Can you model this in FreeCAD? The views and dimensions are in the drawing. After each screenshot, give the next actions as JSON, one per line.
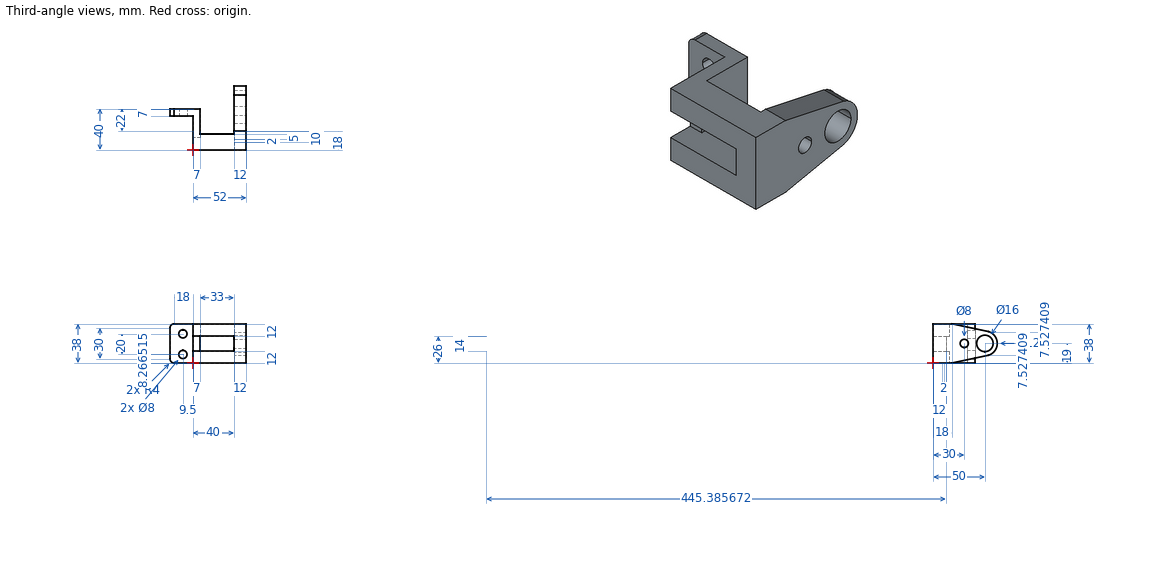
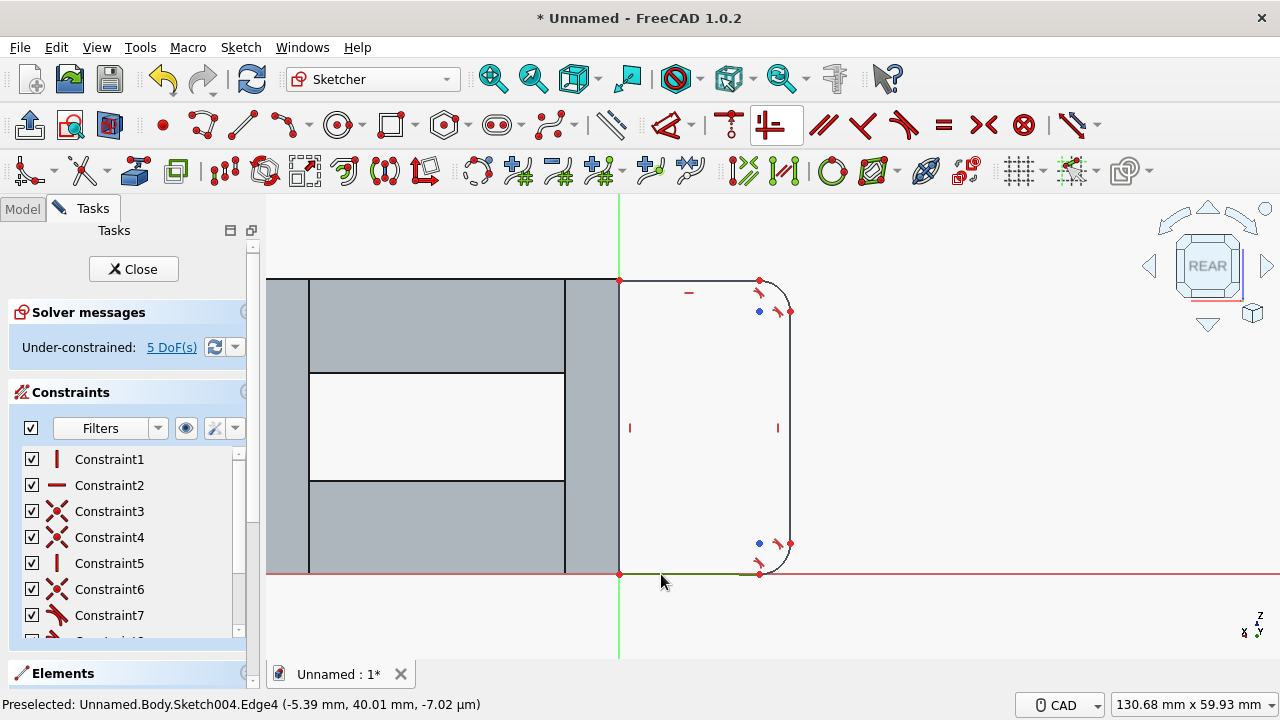
{"action": "key", "text": "h"}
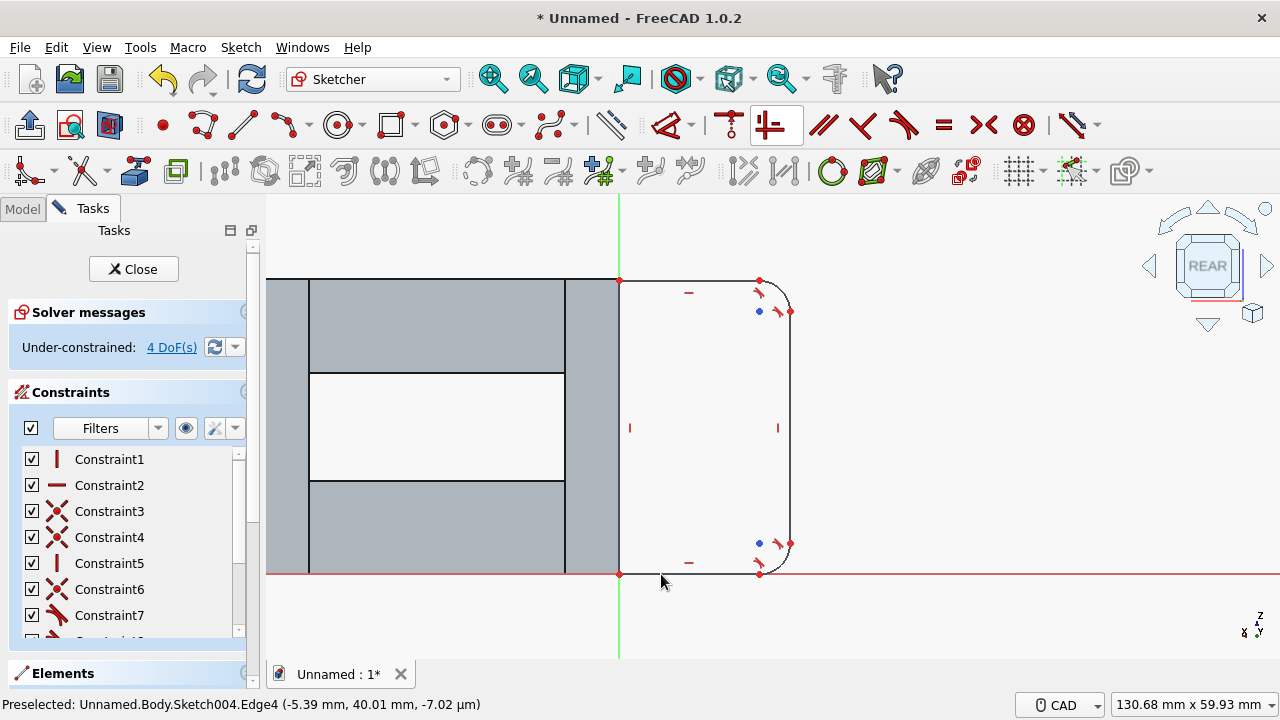
{"action": "left_click", "coordinate": [787, 298]}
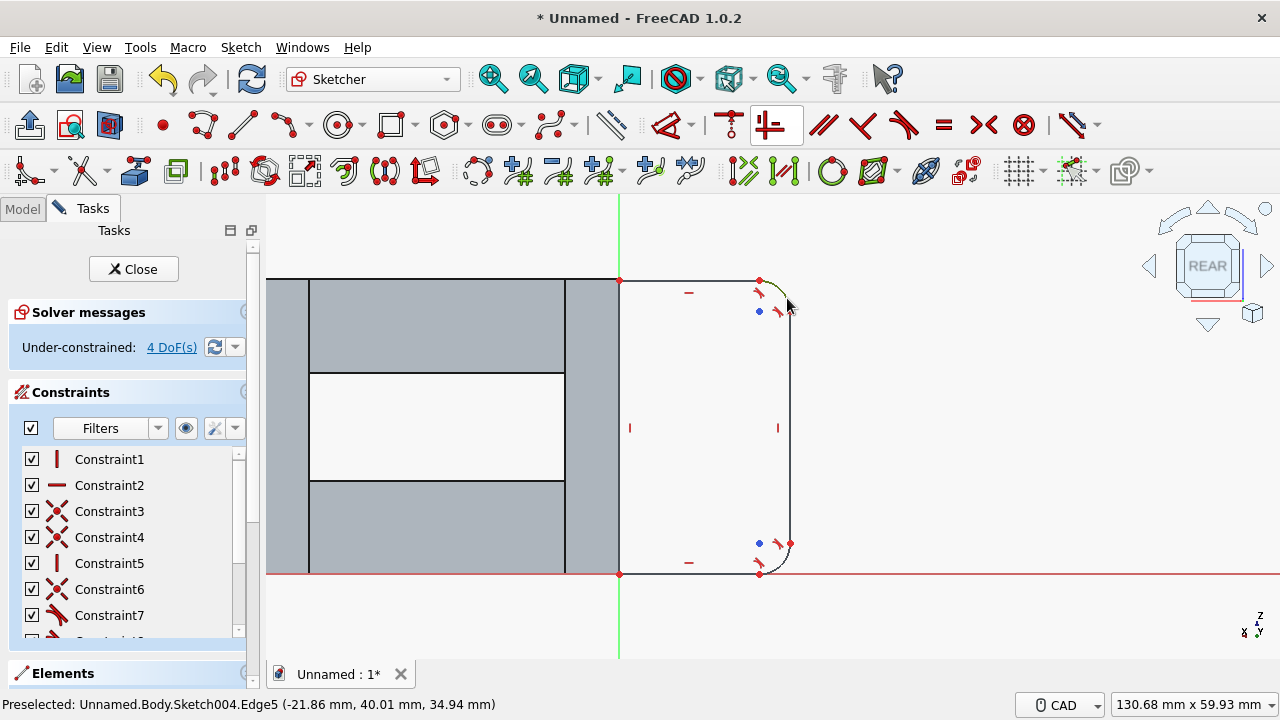
{"action": "left_click", "coordinate": [773, 571]}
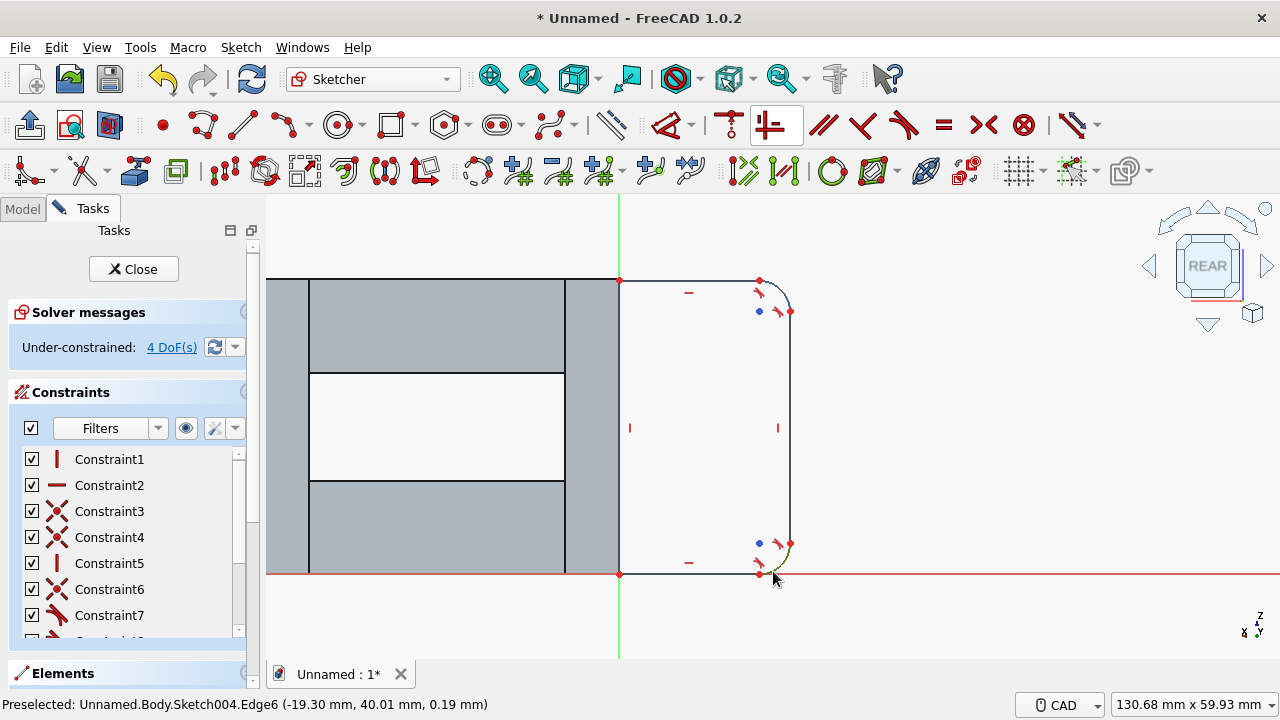
{"action": "left_click", "coordinate": [944, 126]}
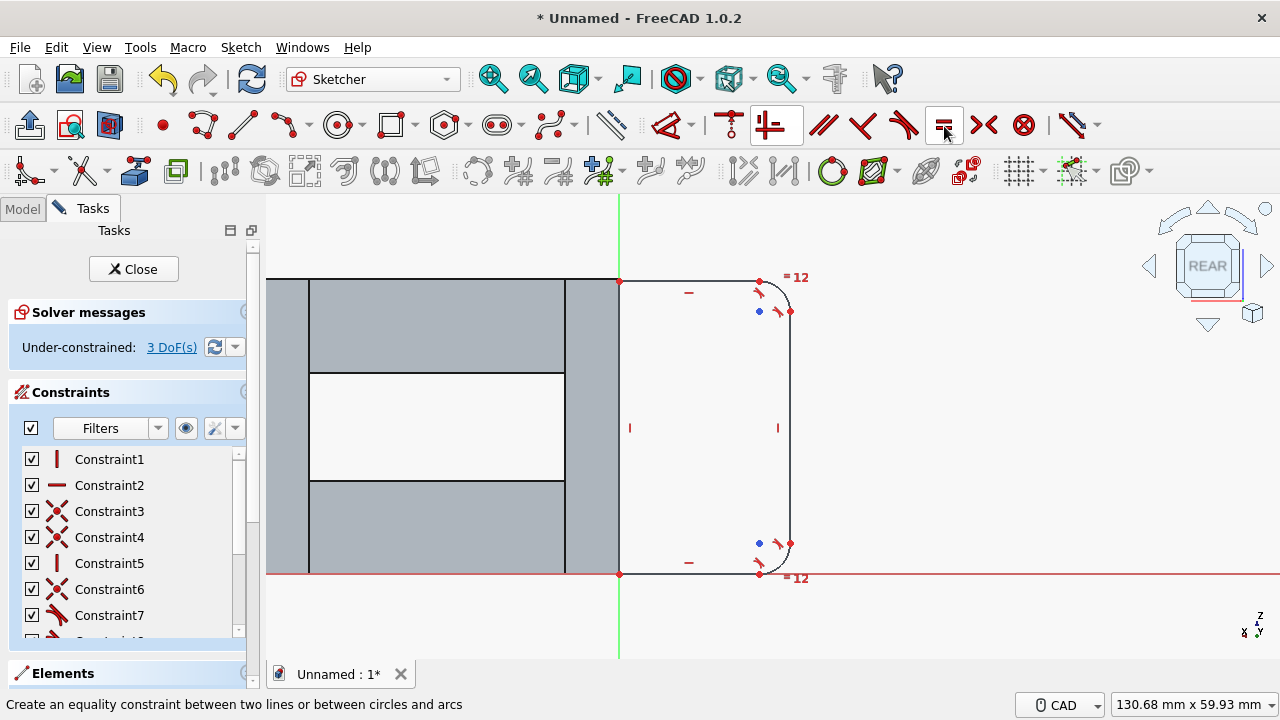
{"action": "left_click", "coordinate": [666, 126]}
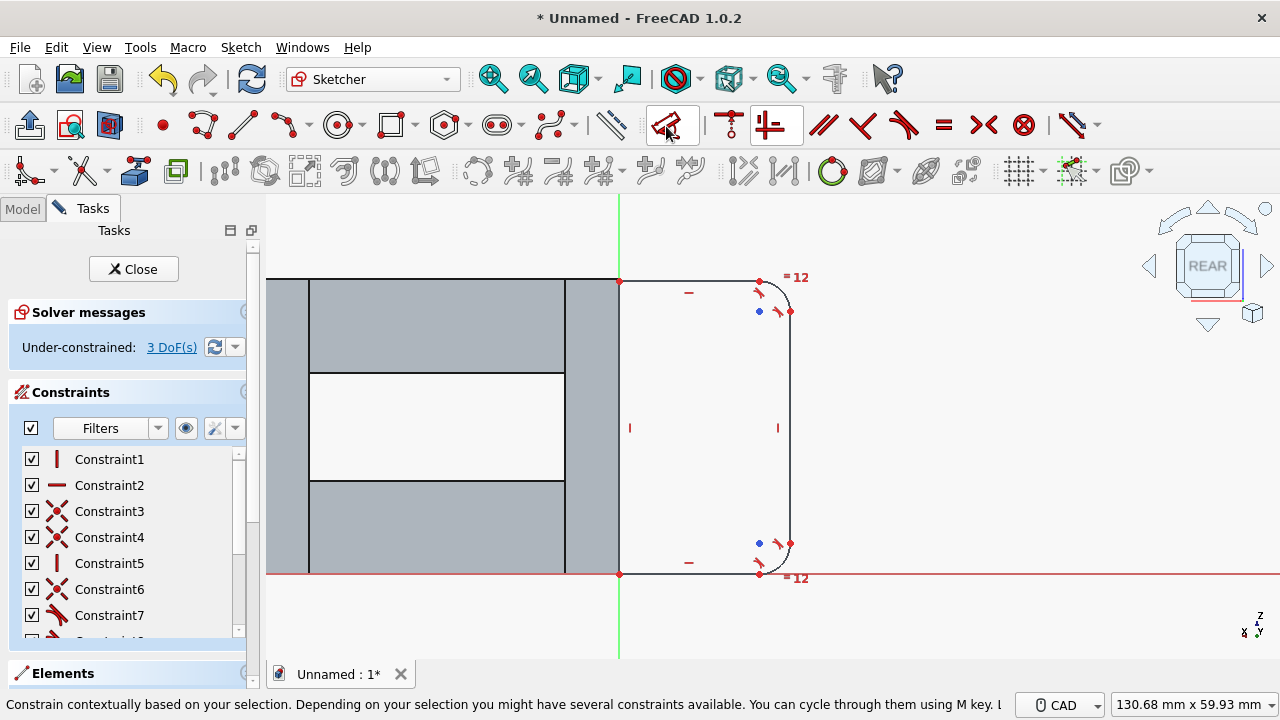
{"action": "scroll", "coordinate": [787, 298], "scroll_direction": "up", "scroll_amount": 2}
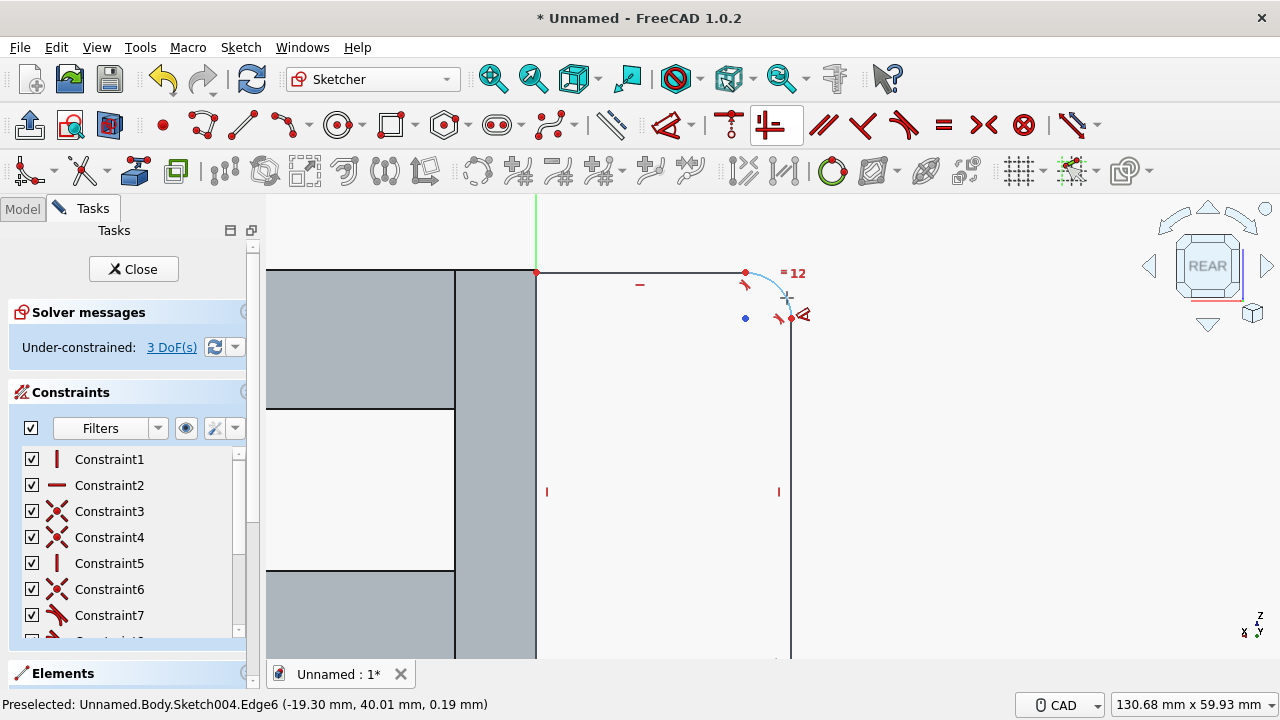
{"action": "left_click", "coordinate": [786, 298]}
{"action": "left_click", "coordinate": [815, 283]}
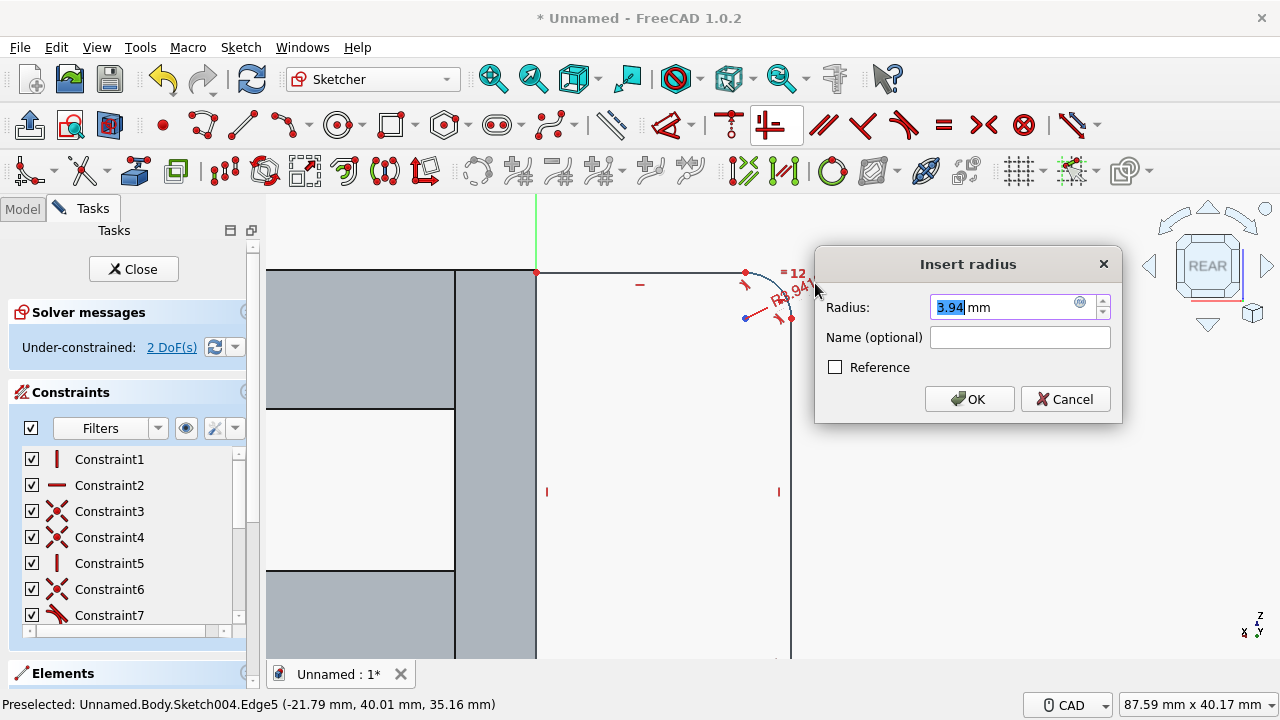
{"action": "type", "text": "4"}
{"action": "key", "text": "Return"}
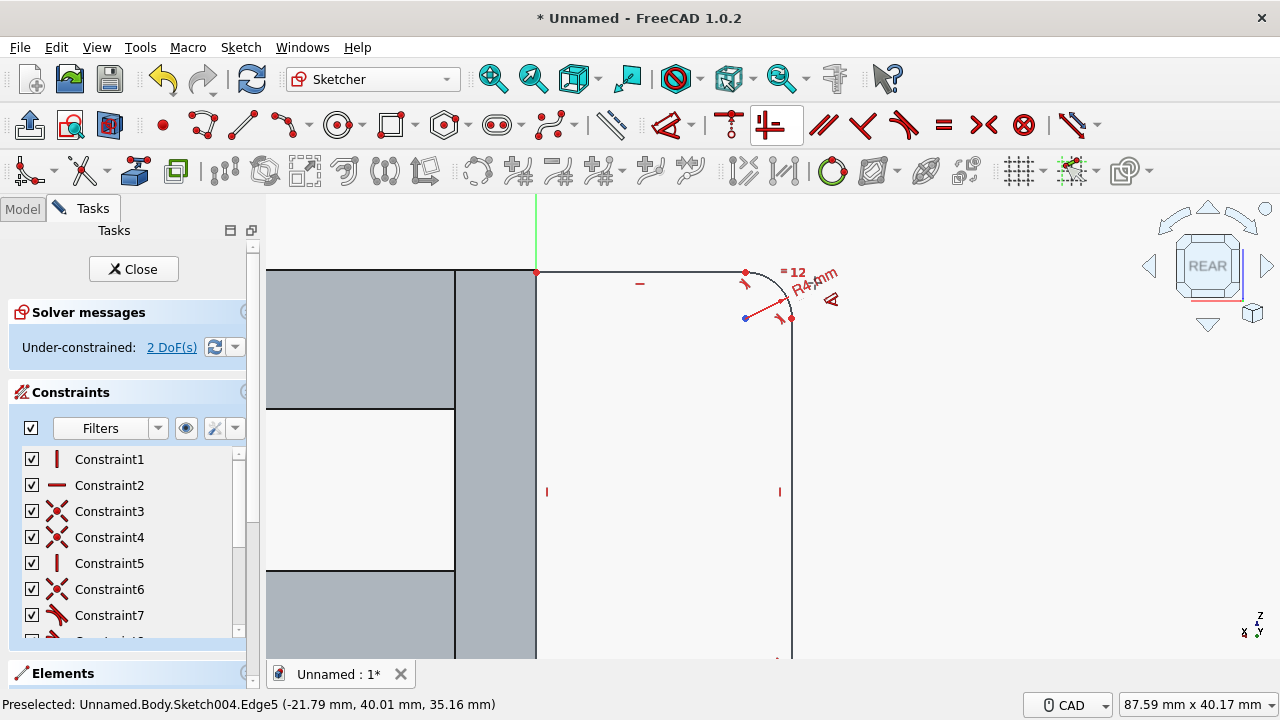
{"action": "left_click", "coordinate": [792, 560]}
{"action": "left_click", "coordinate": [826, 475]}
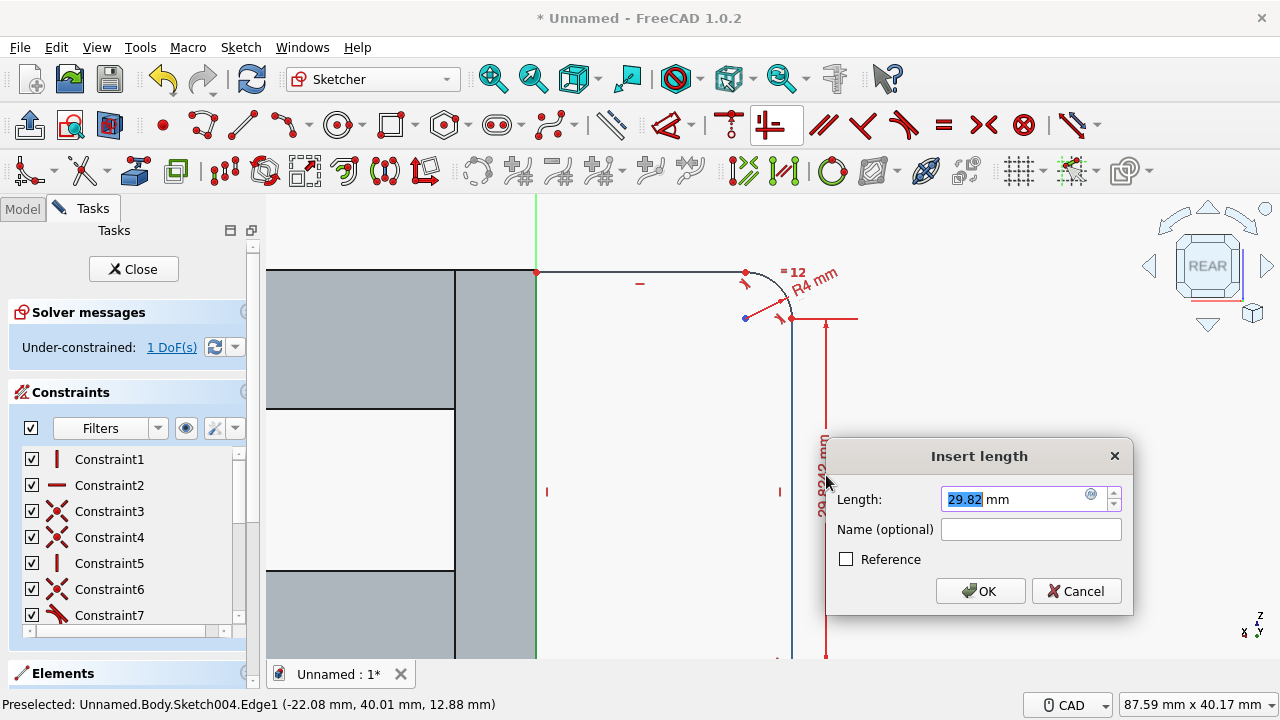
{"action": "type", "text": "30"}
{"action": "key", "text": "Return"}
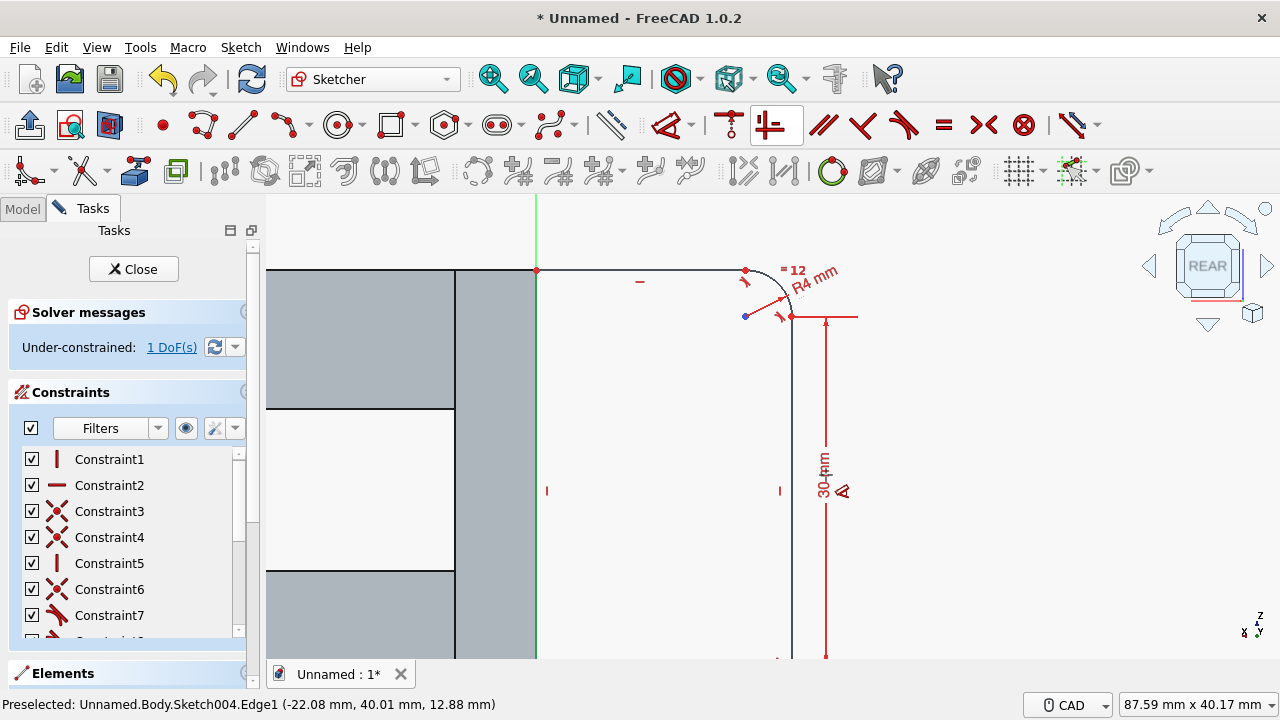
{"action": "left_click", "coordinate": [683, 270]}
{"action": "left_click", "coordinate": [641, 236]}